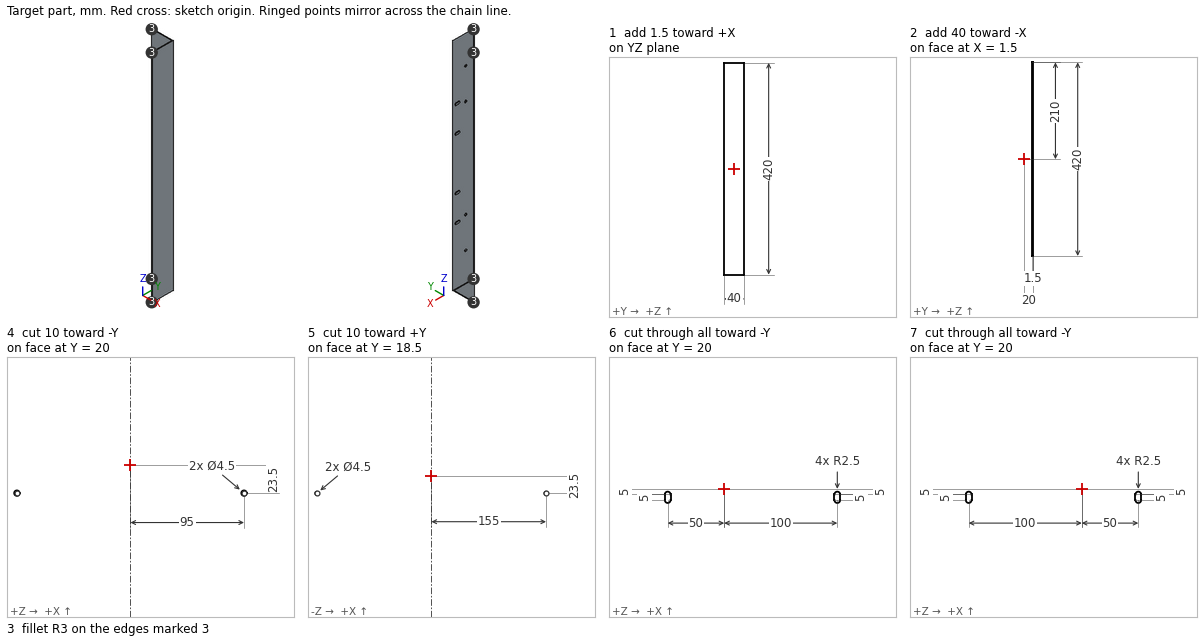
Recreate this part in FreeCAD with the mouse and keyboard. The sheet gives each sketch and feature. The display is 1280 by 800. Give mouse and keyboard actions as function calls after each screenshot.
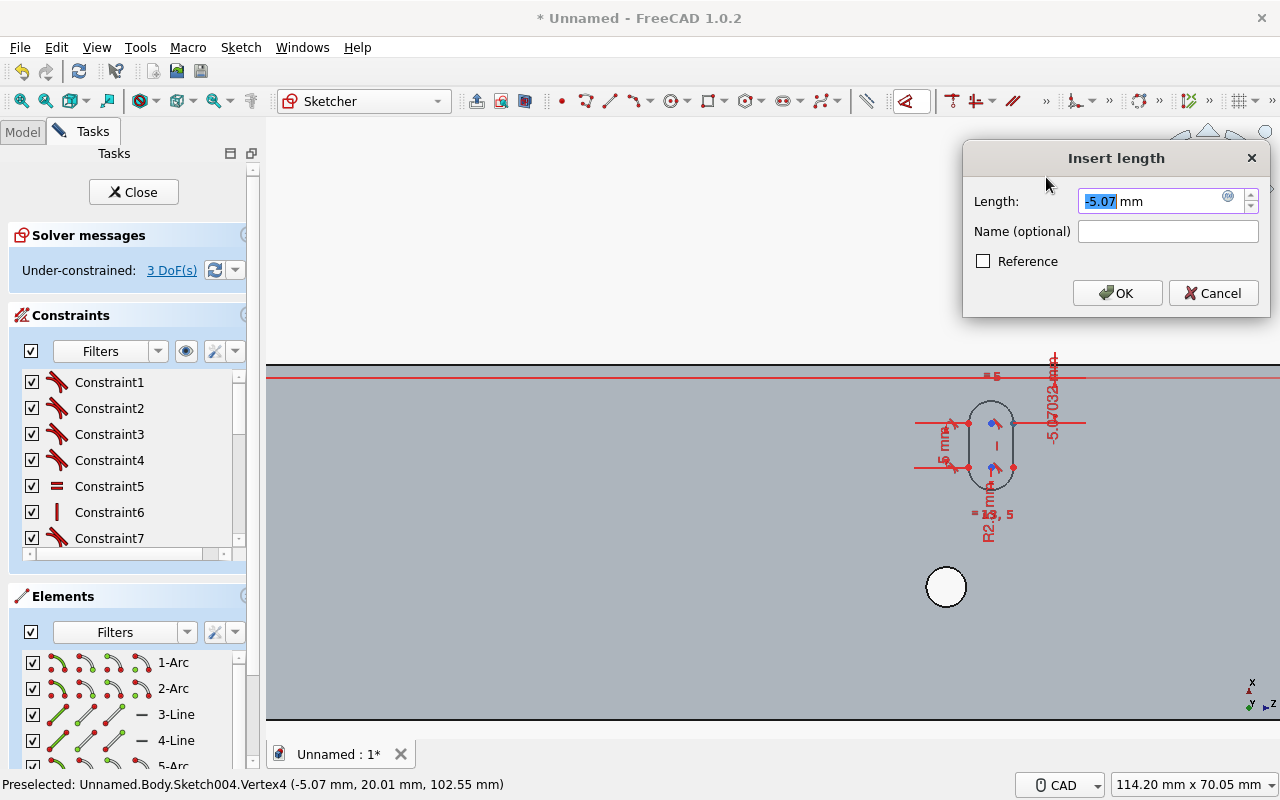
text(-5)
key(Return)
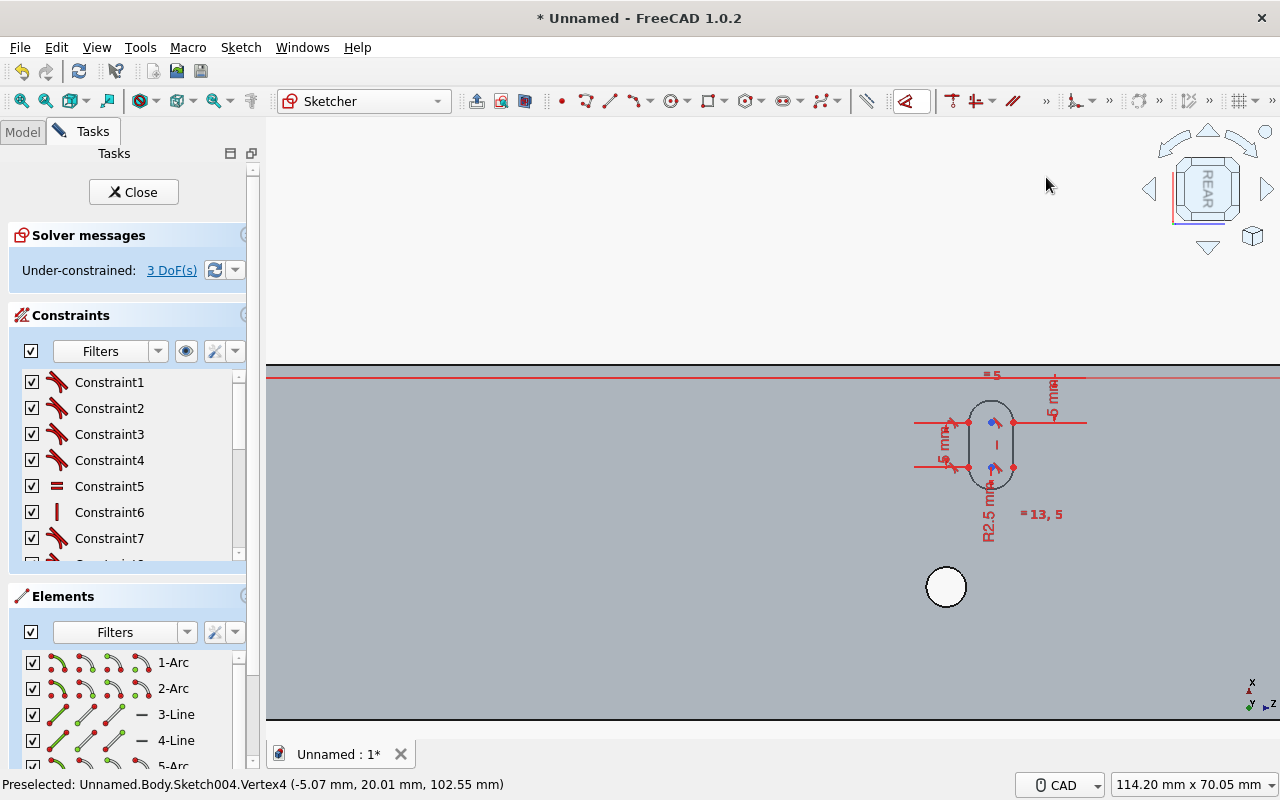
scroll(1014, 423, down, 4)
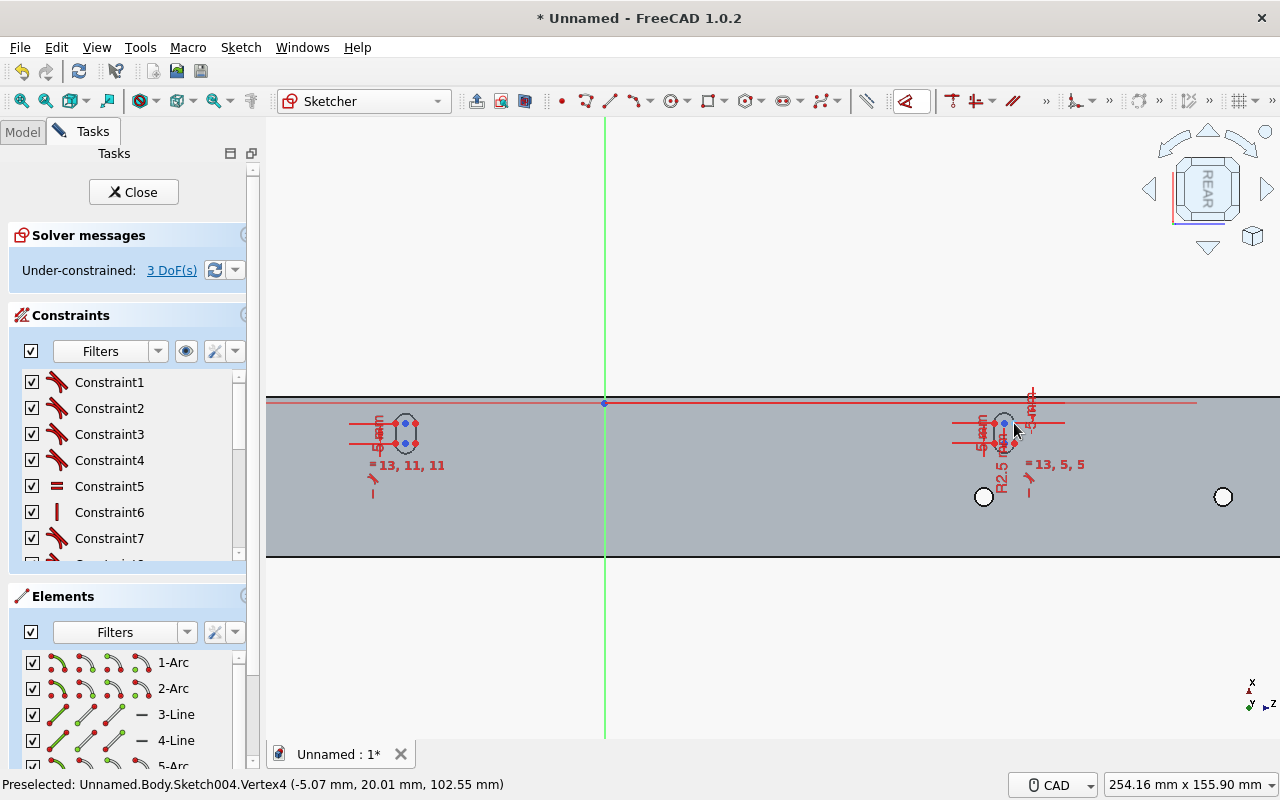
scroll(416, 424, up, 4)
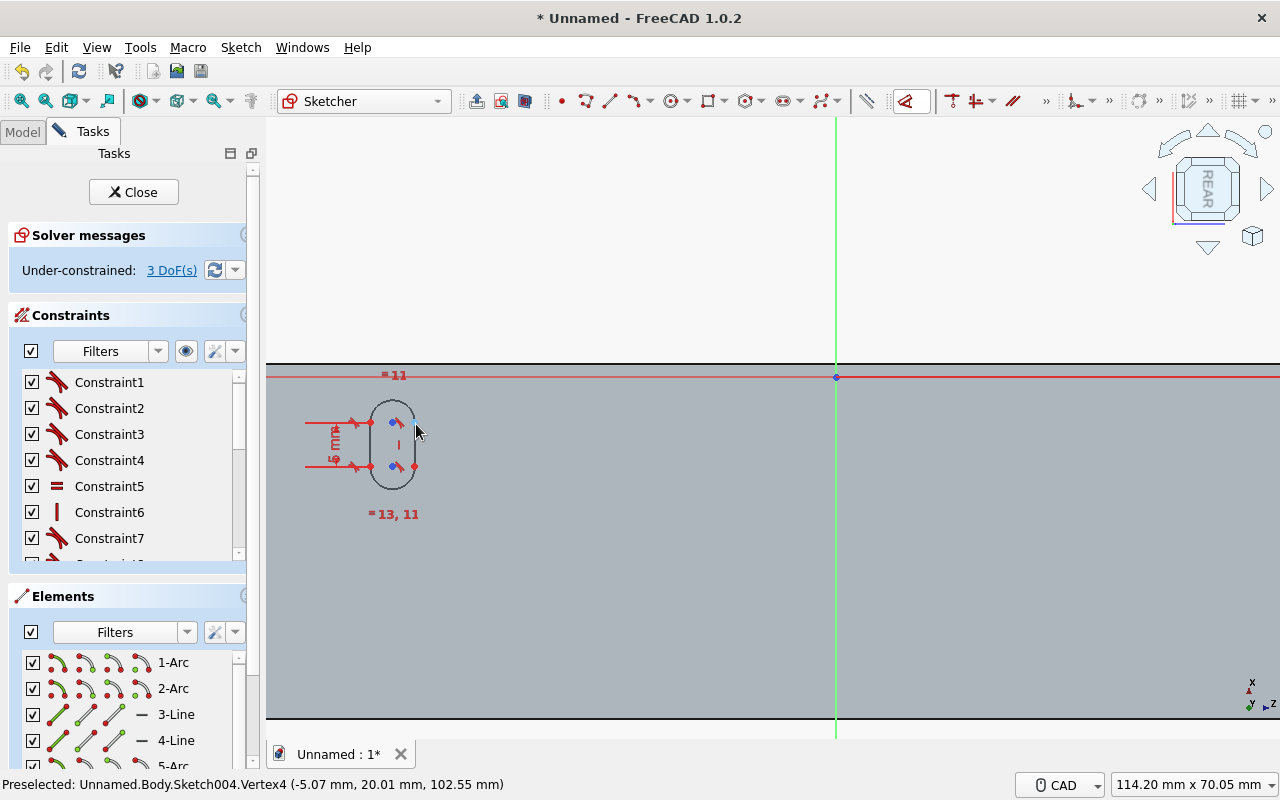
click(415, 423)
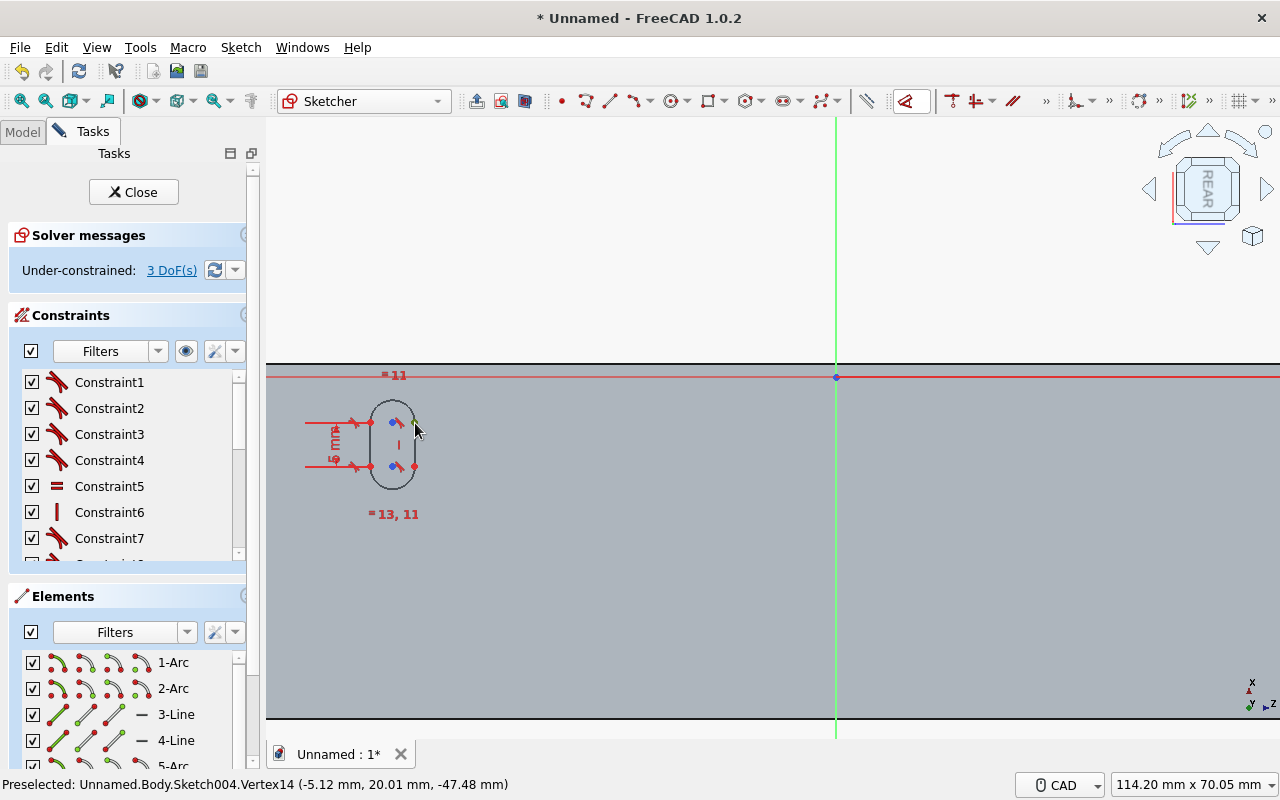
click(924, 102)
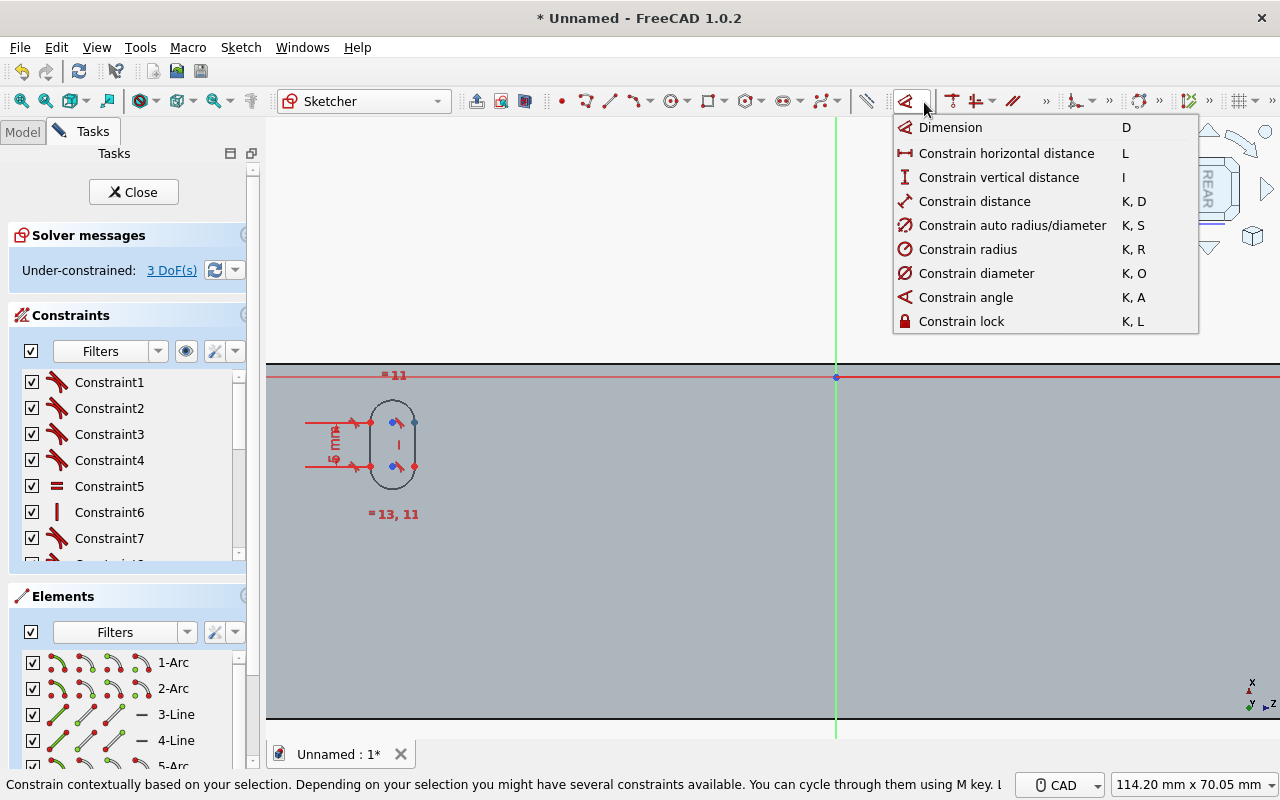
click(1046, 177)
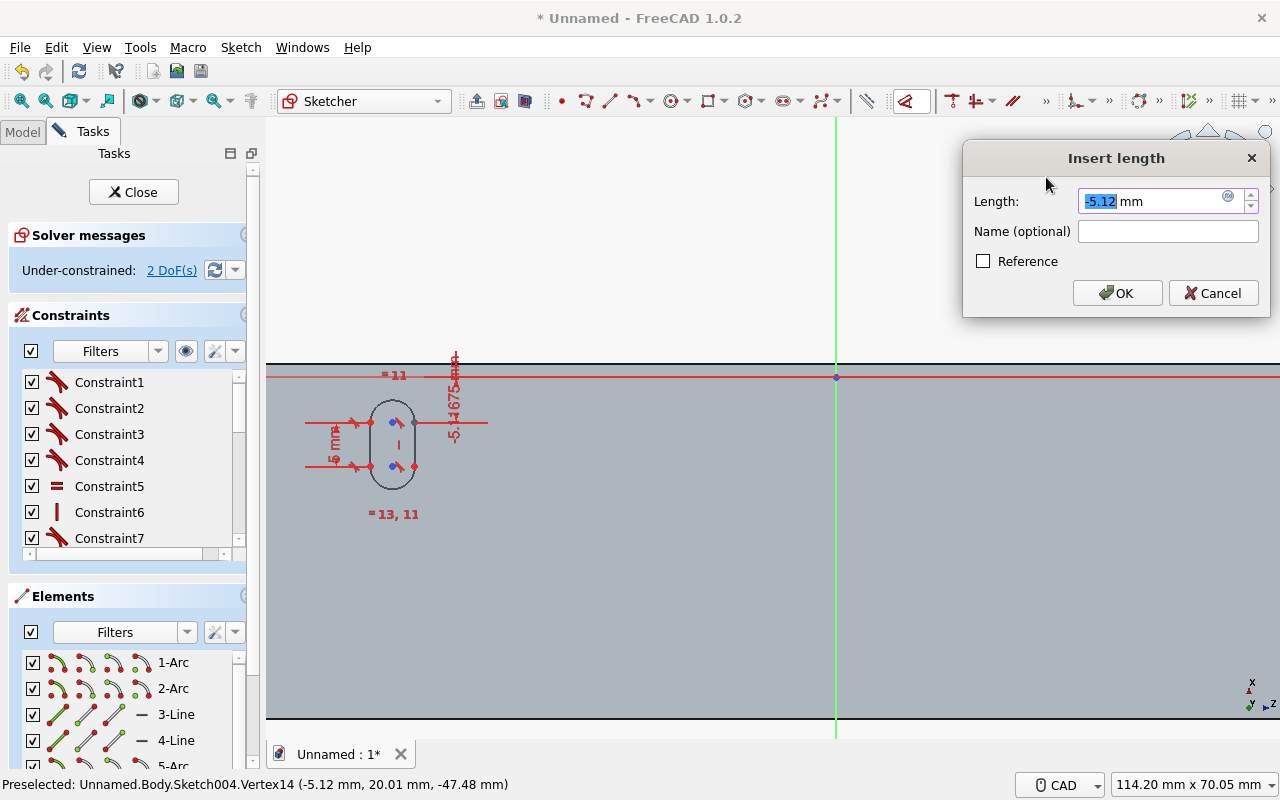
text(-5)
key(Return)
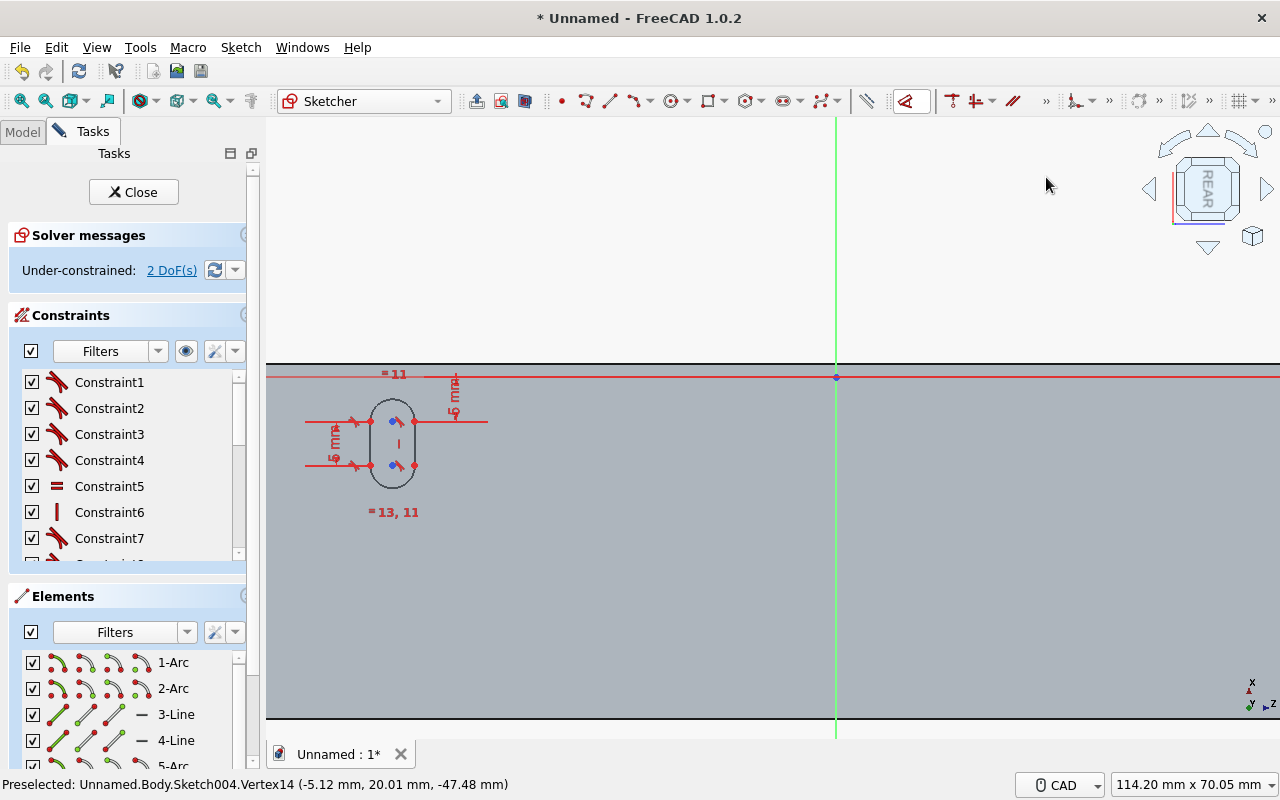
click(393, 466)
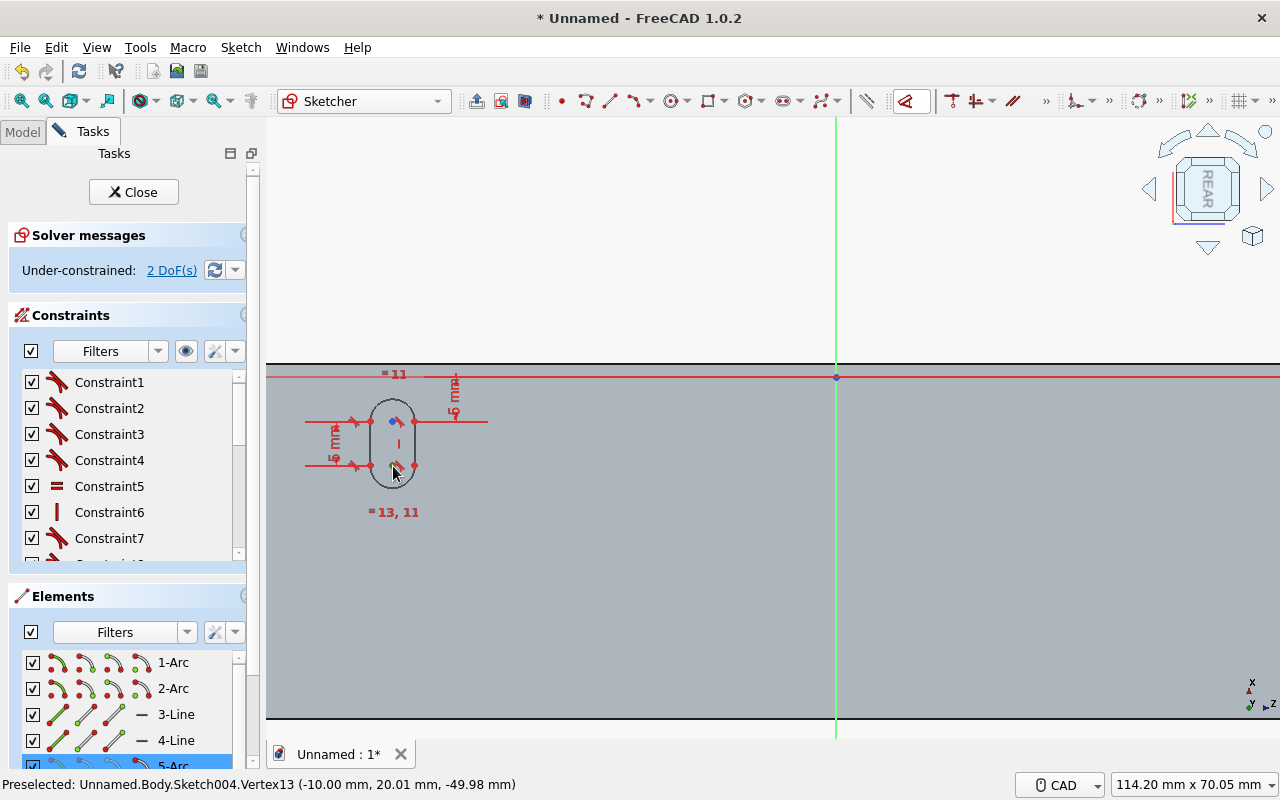
key(l)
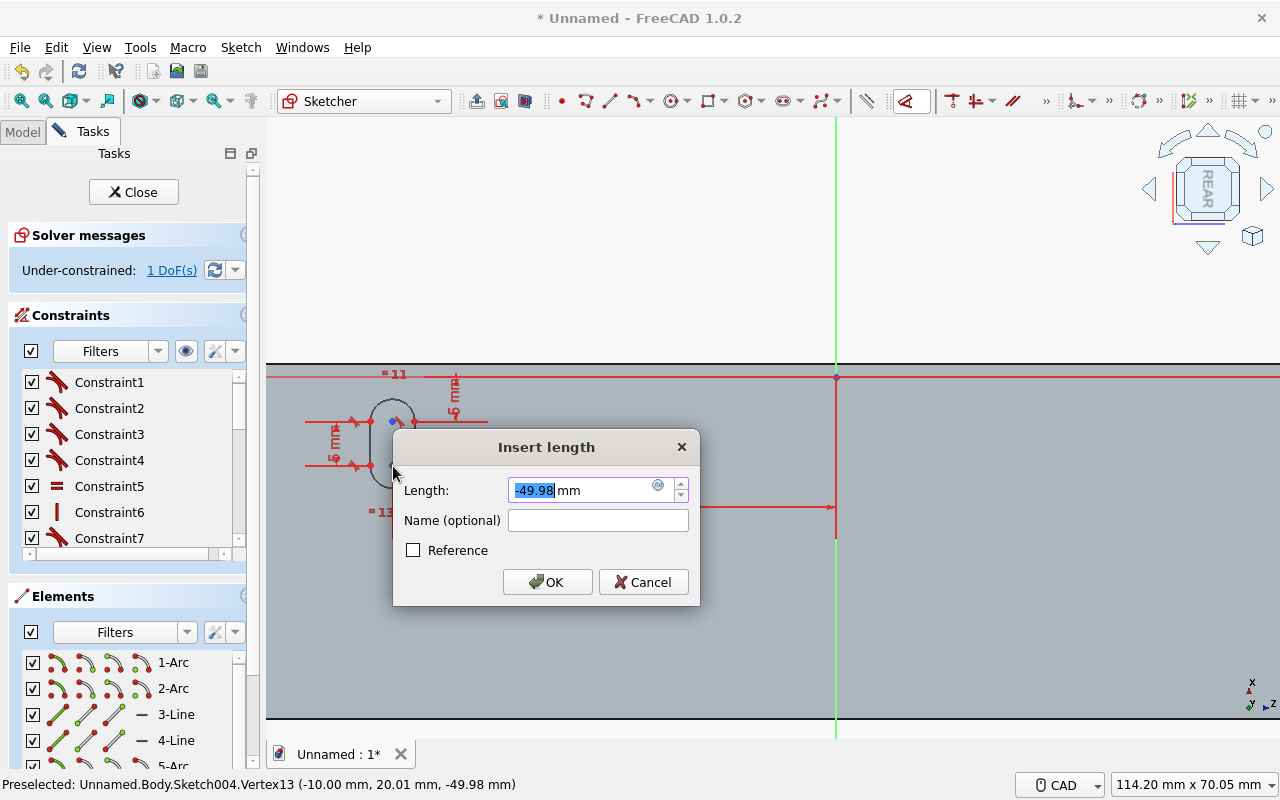
text(-50)
key(Return)